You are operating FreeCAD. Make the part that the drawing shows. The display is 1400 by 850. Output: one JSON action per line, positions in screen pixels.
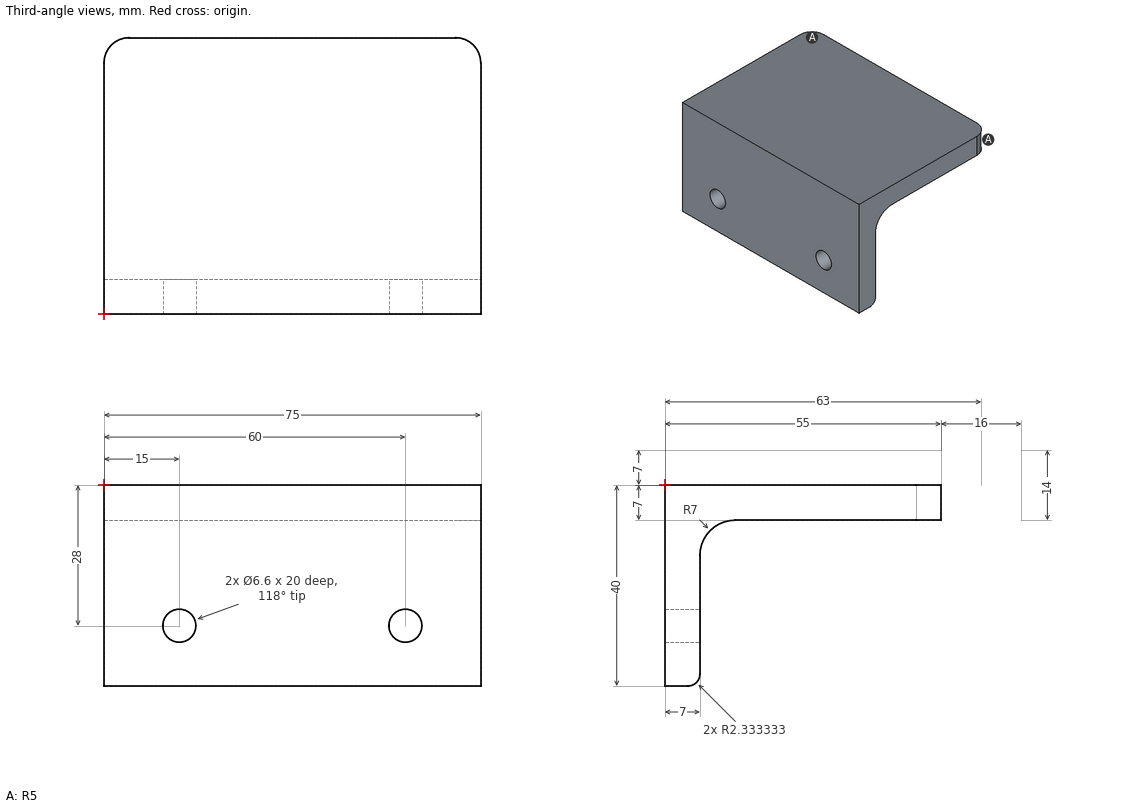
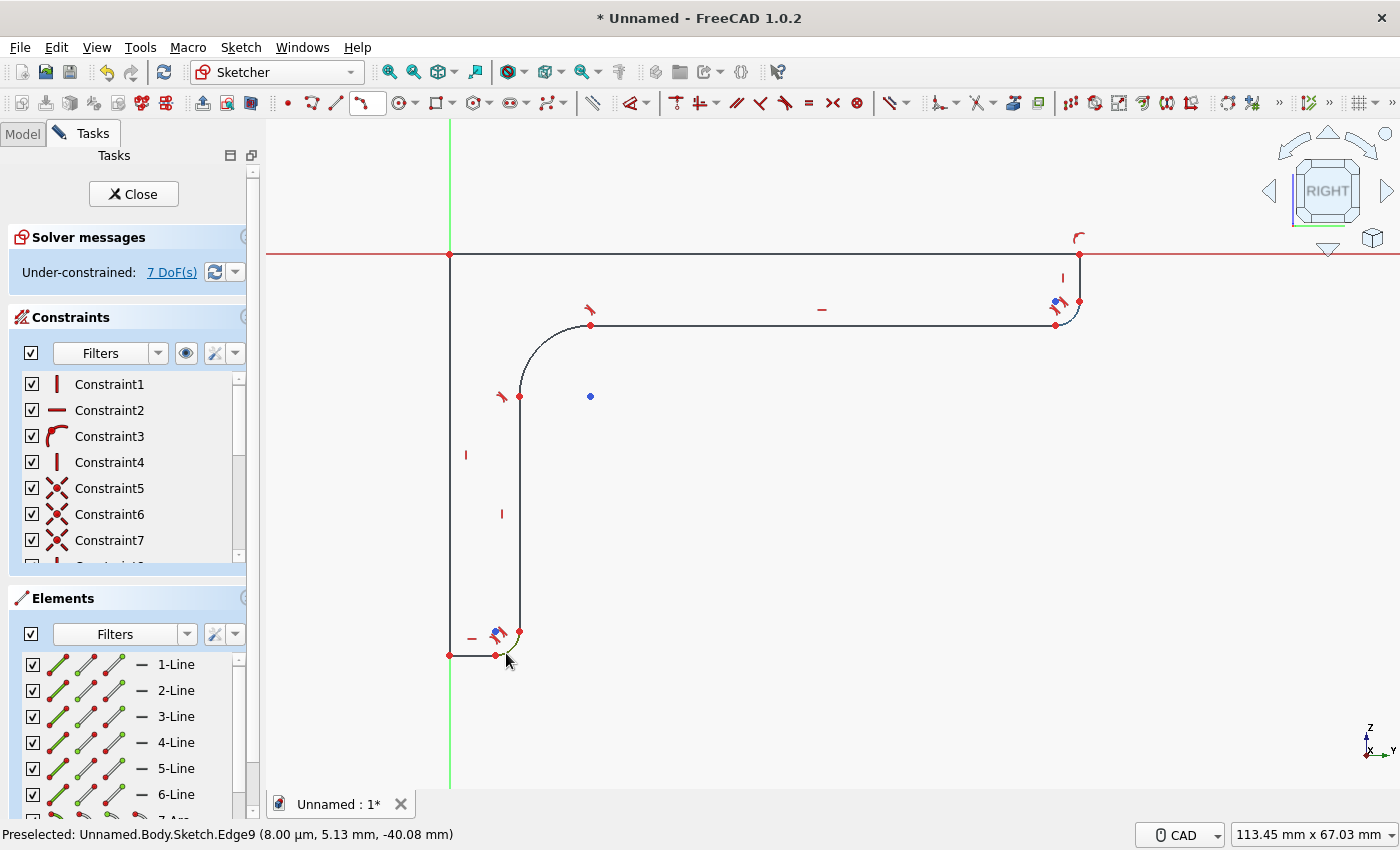
{"action": "left_click", "coordinate": [810, 104]}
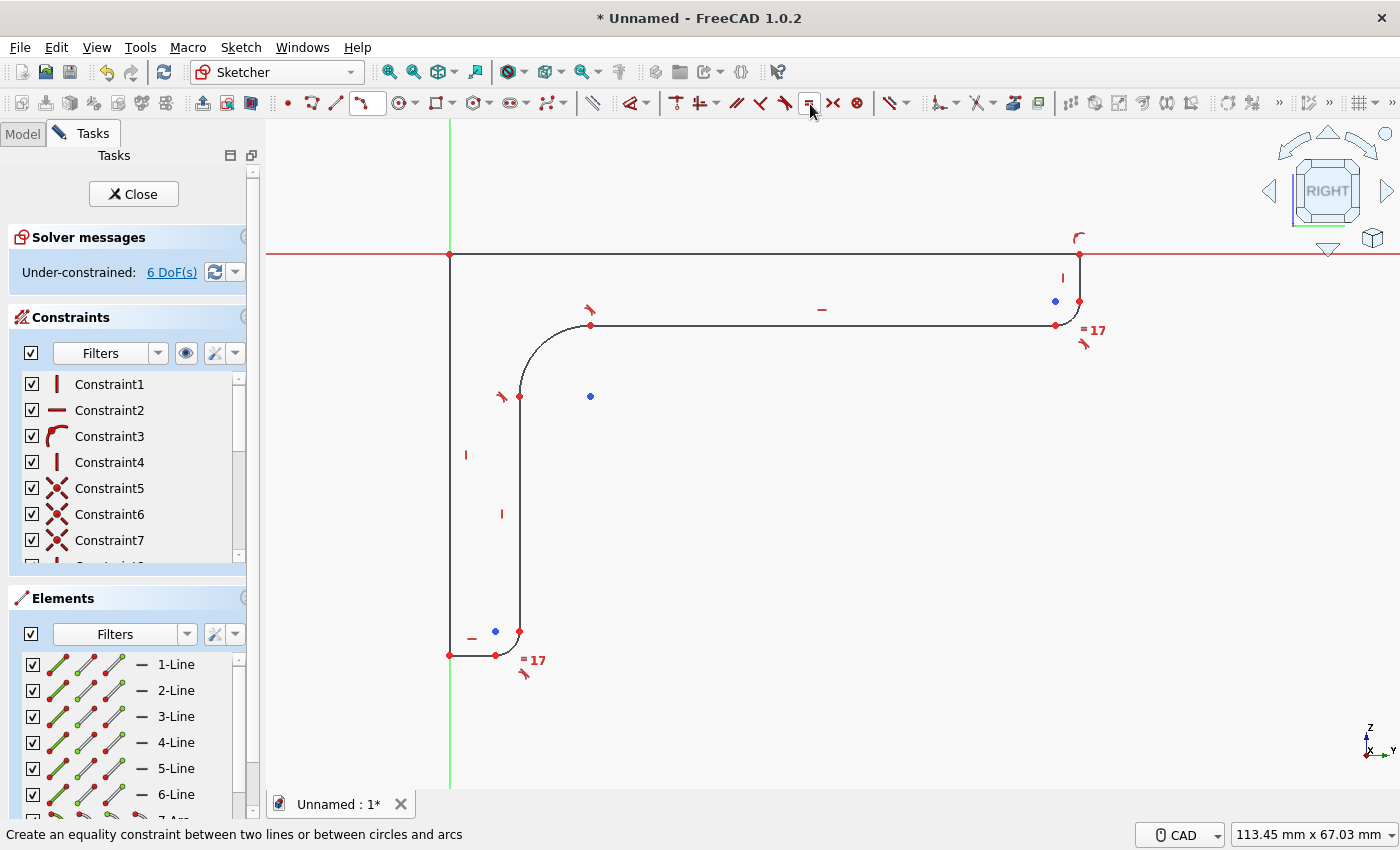
{"action": "left_click", "coordinate": [630, 104]}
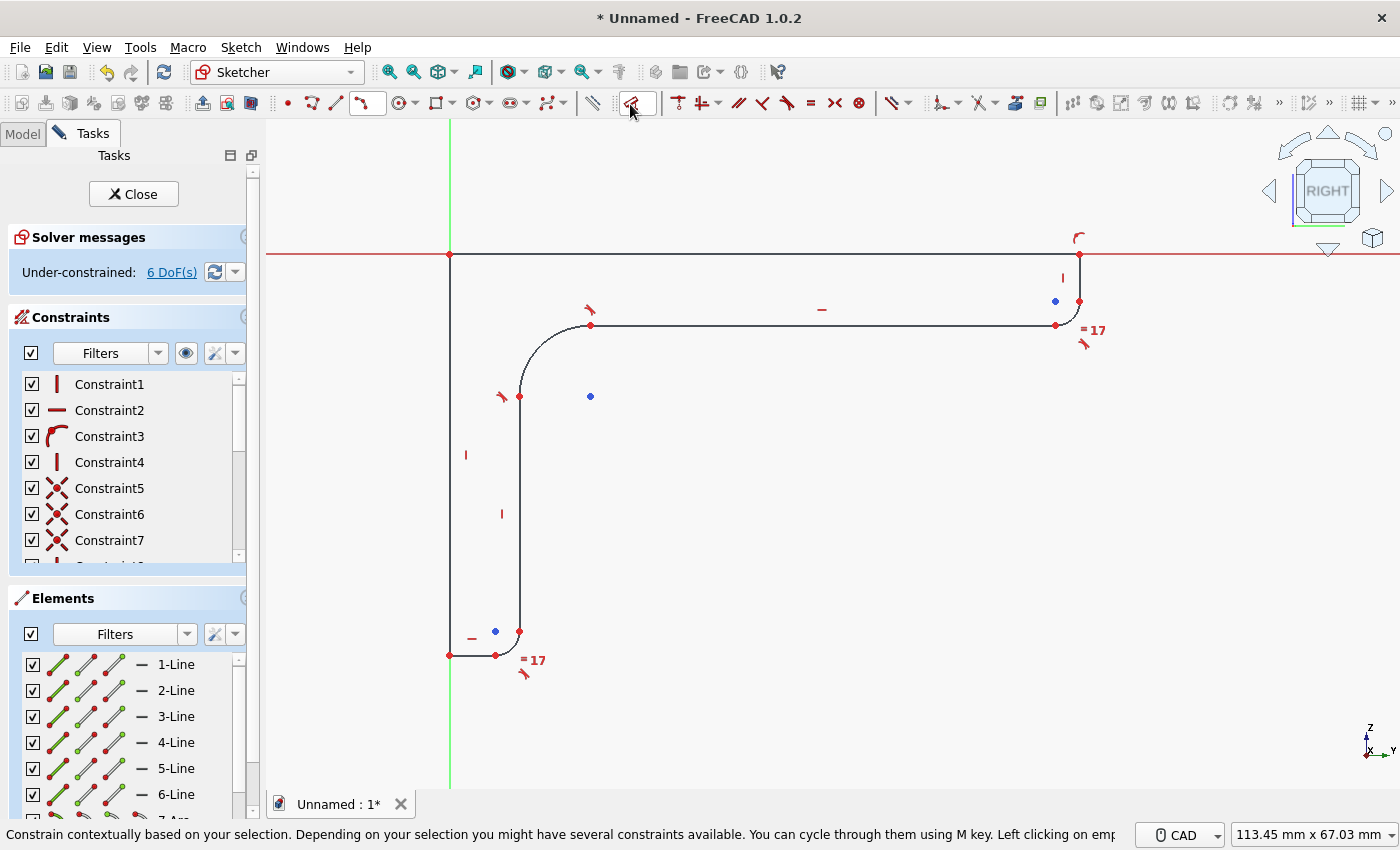
{"action": "left_click", "coordinate": [558, 333]}
{"action": "left_click", "coordinate": [544, 304]}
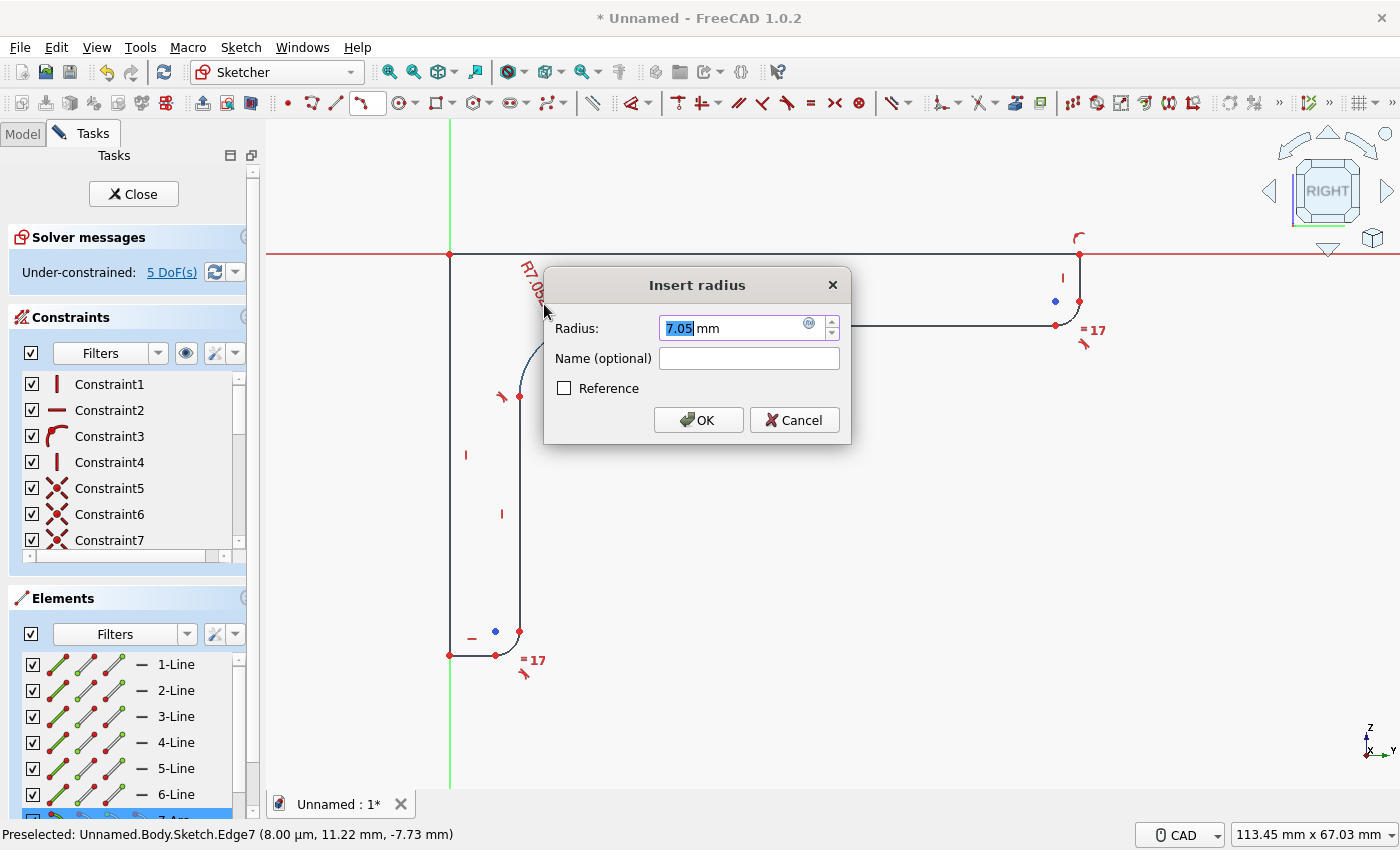
{"action": "type", "text": "7"}
{"action": "key", "text": "Return"}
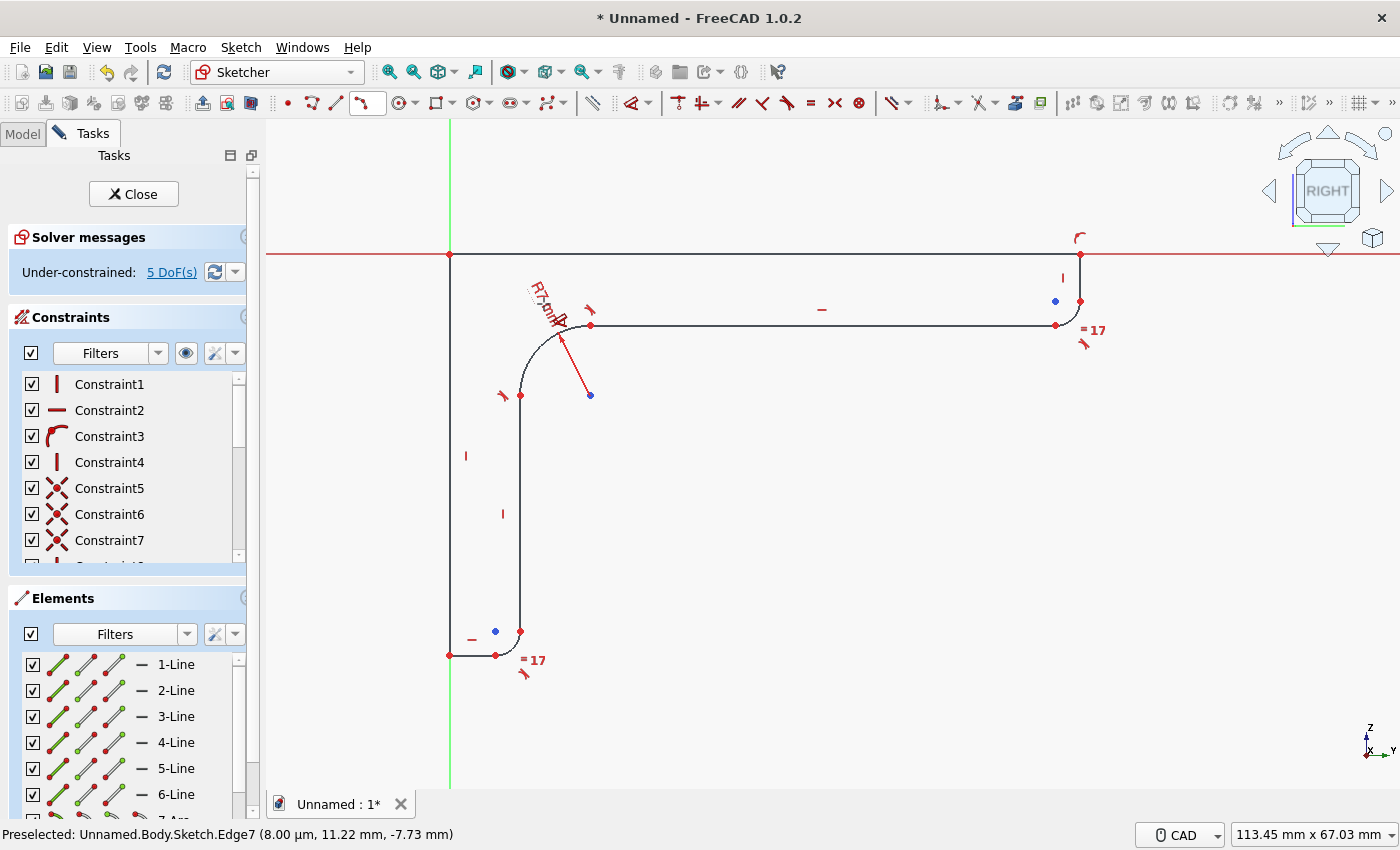
{"action": "scroll", "coordinate": [1067, 323], "scroll_direction": "up", "scroll_amount": 3}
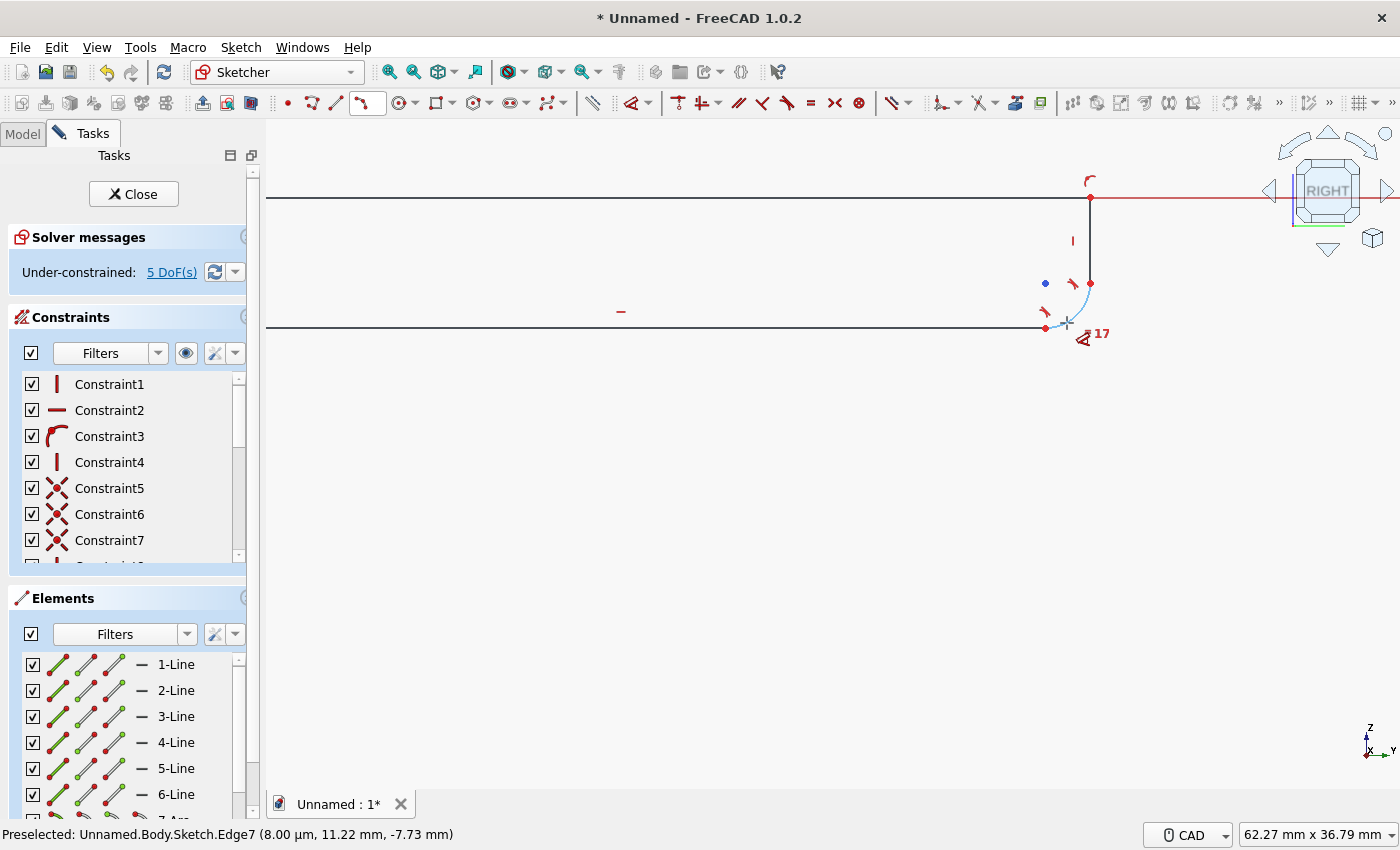
{"action": "left_click", "coordinate": [1066, 323]}
{"action": "left_click", "coordinate": [1081, 351]}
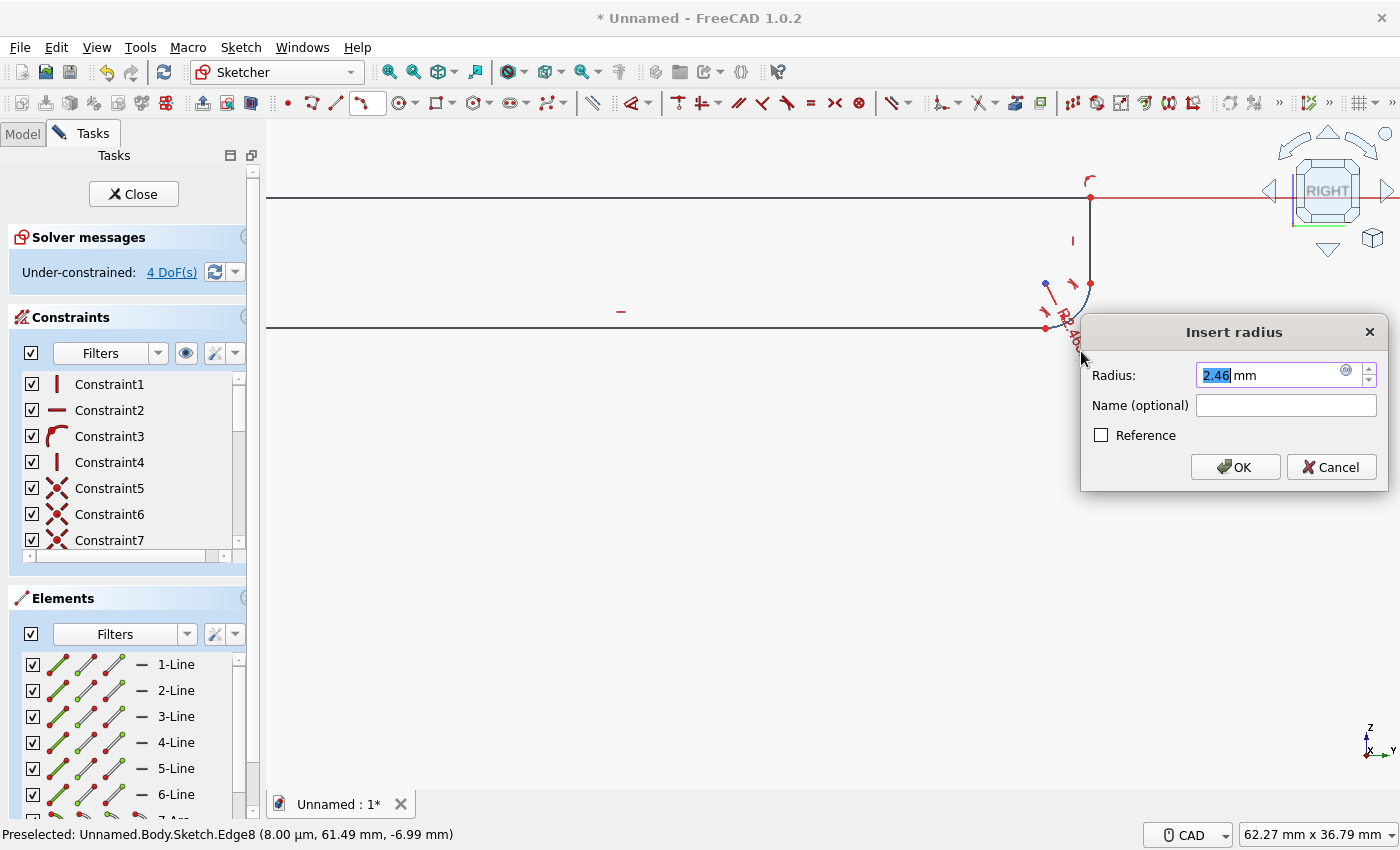
{"action": "type", "text": "2.333333"}
{"action": "key", "text": "Return"}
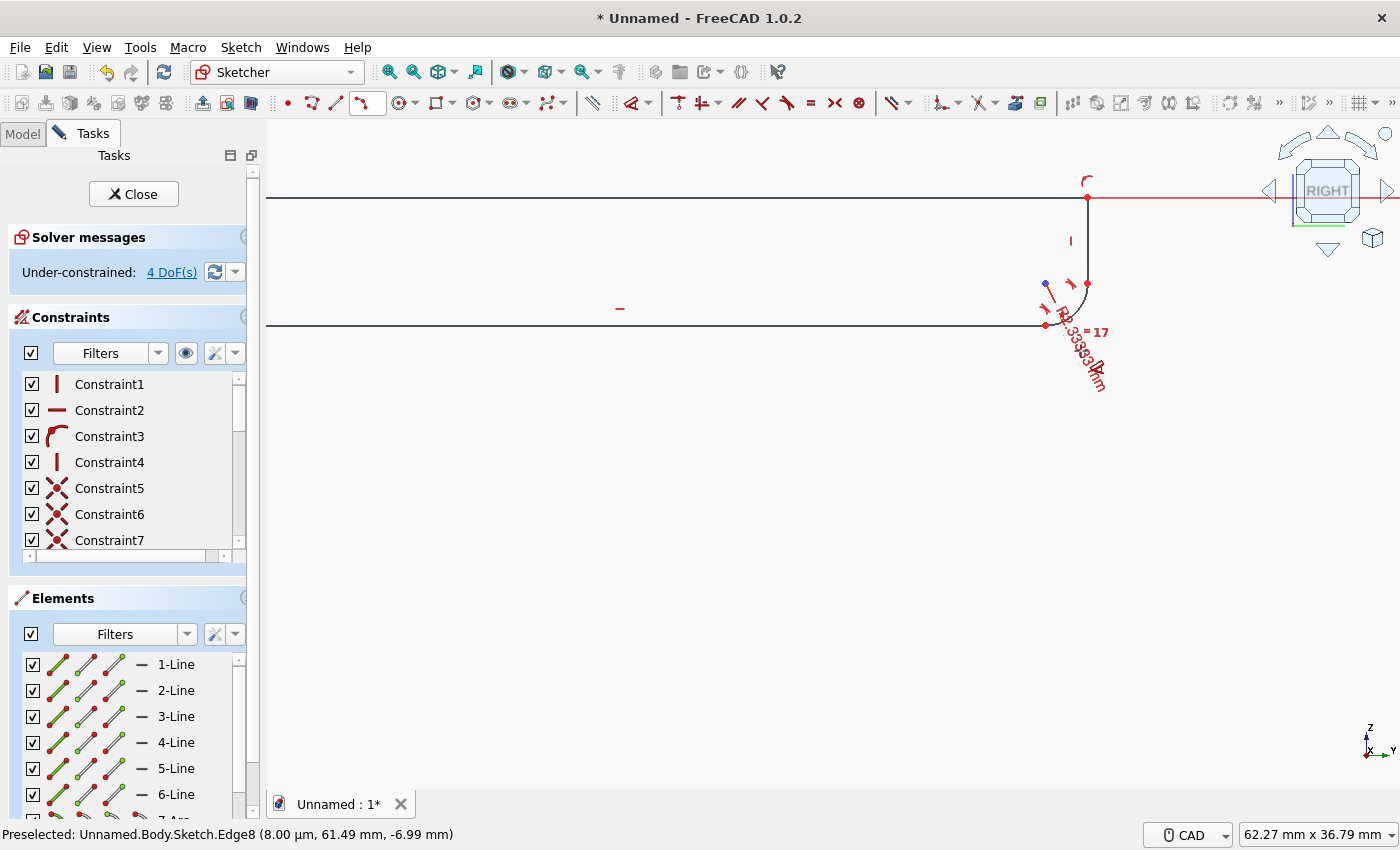
{"action": "left_click", "coordinate": [744, 198]}
{"action": "left_click", "coordinate": [691, 164]}